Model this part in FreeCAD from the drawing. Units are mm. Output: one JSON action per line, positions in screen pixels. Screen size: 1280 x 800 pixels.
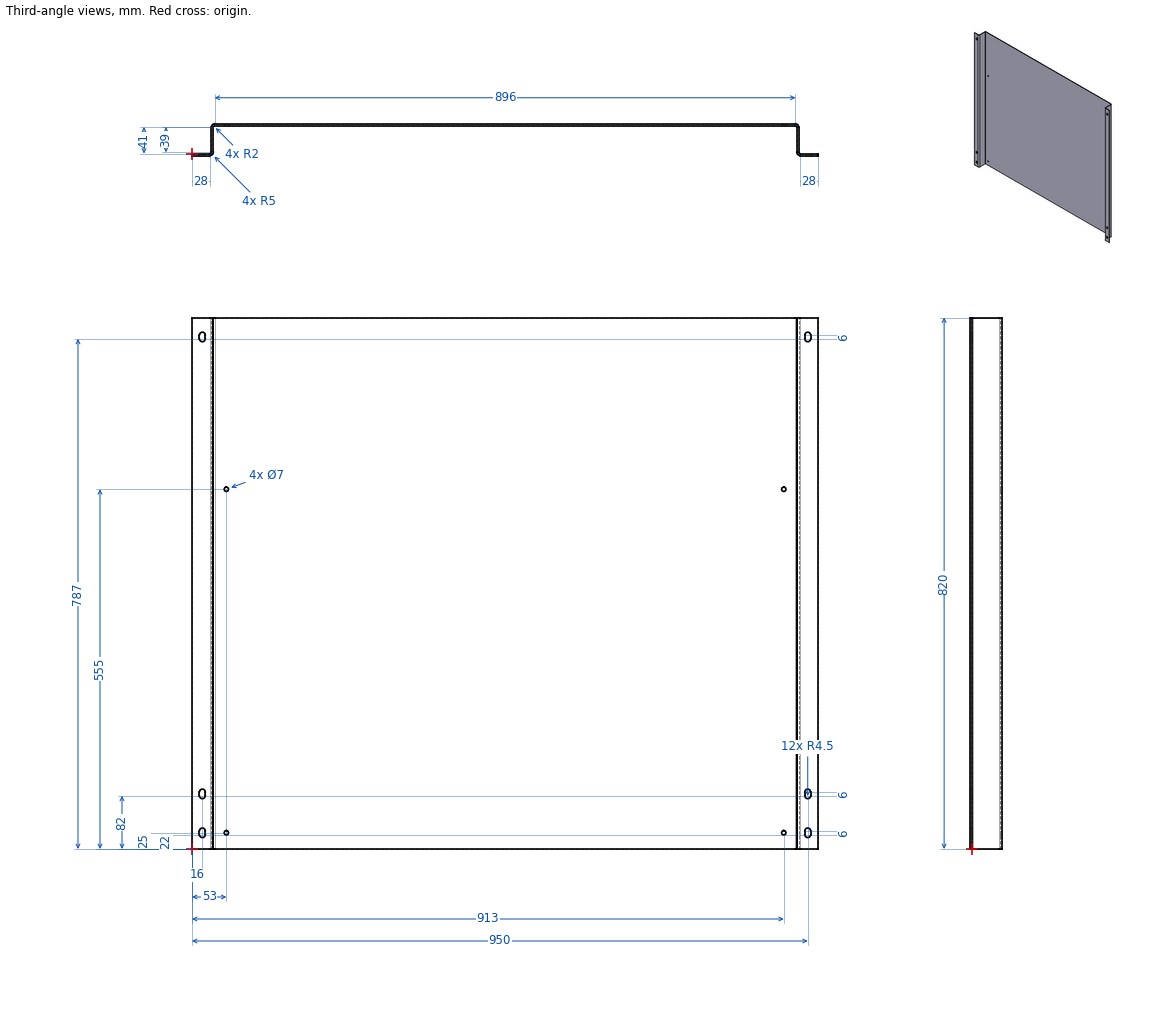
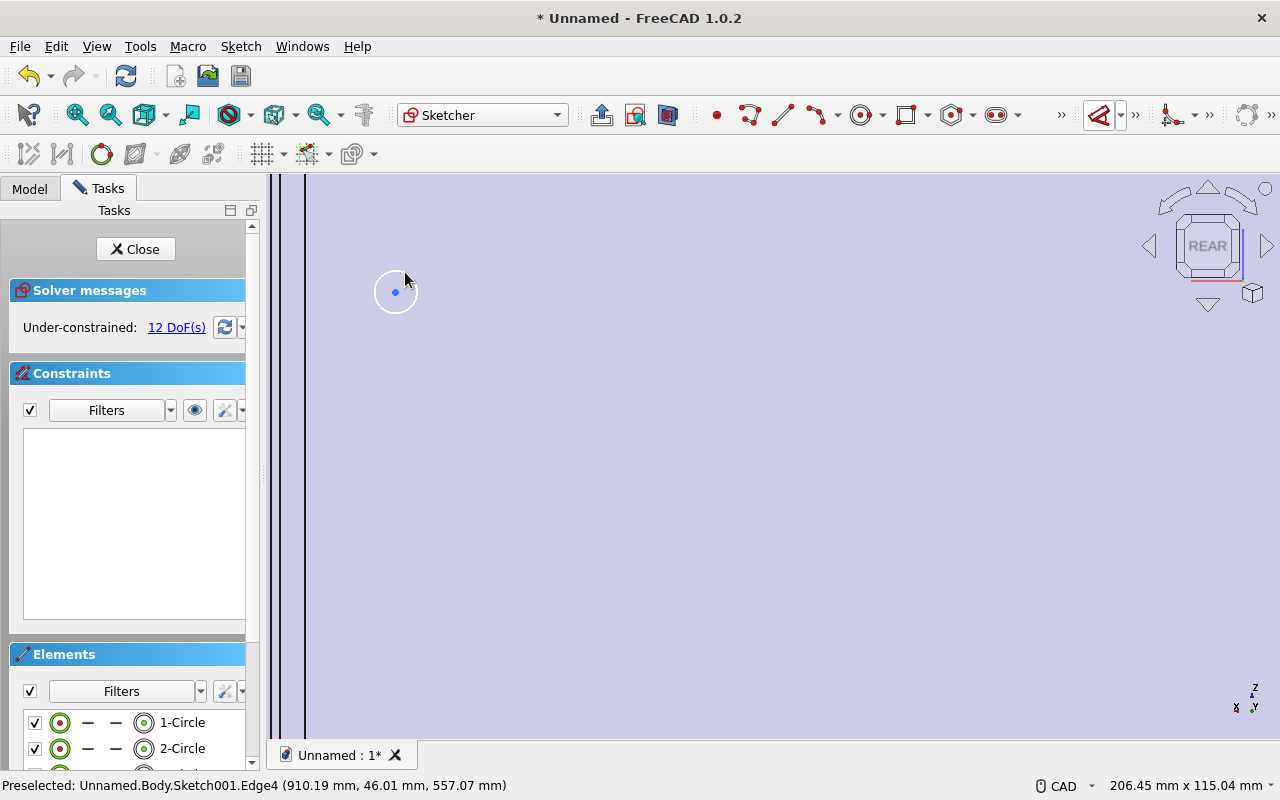
{"action": "scroll", "coordinate": [404, 271], "scroll_direction": "down", "scroll_amount": 10}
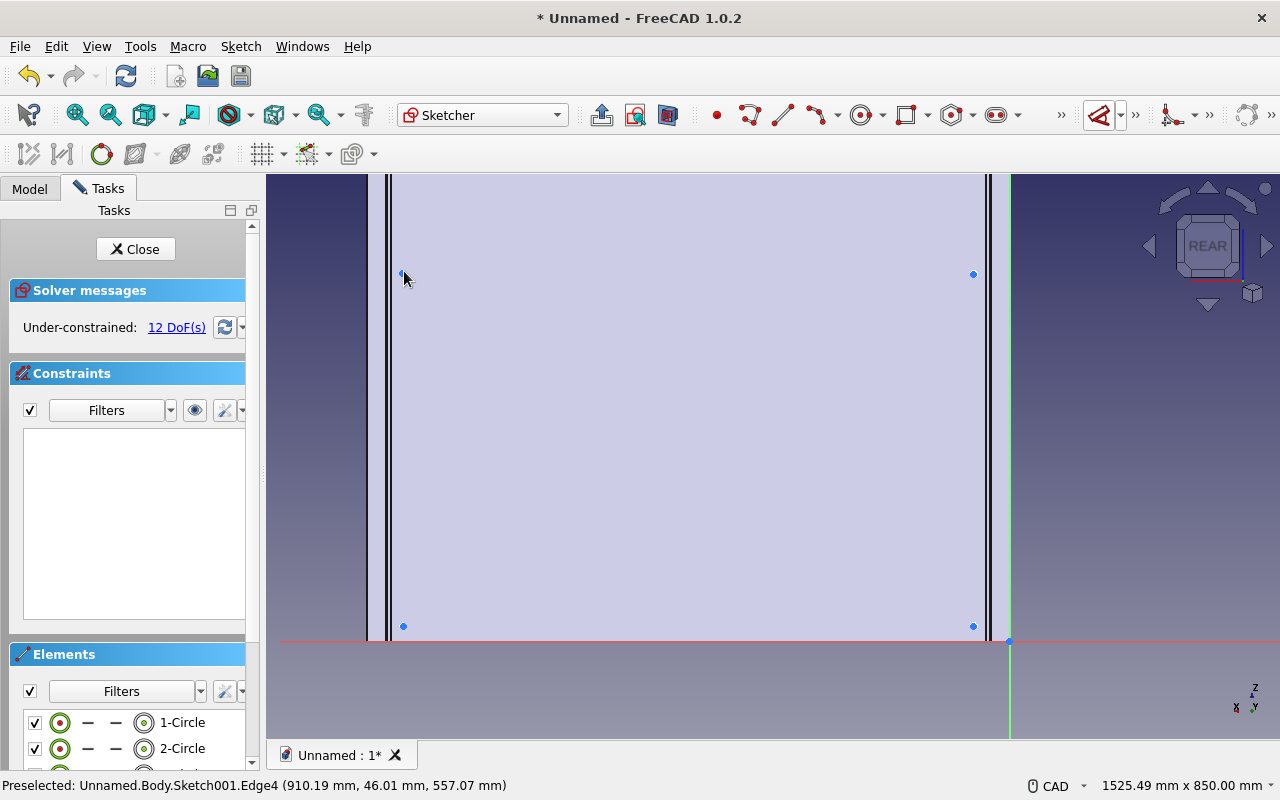
{"action": "scroll", "coordinate": [976, 272], "scroll_direction": "up", "scroll_amount": 8}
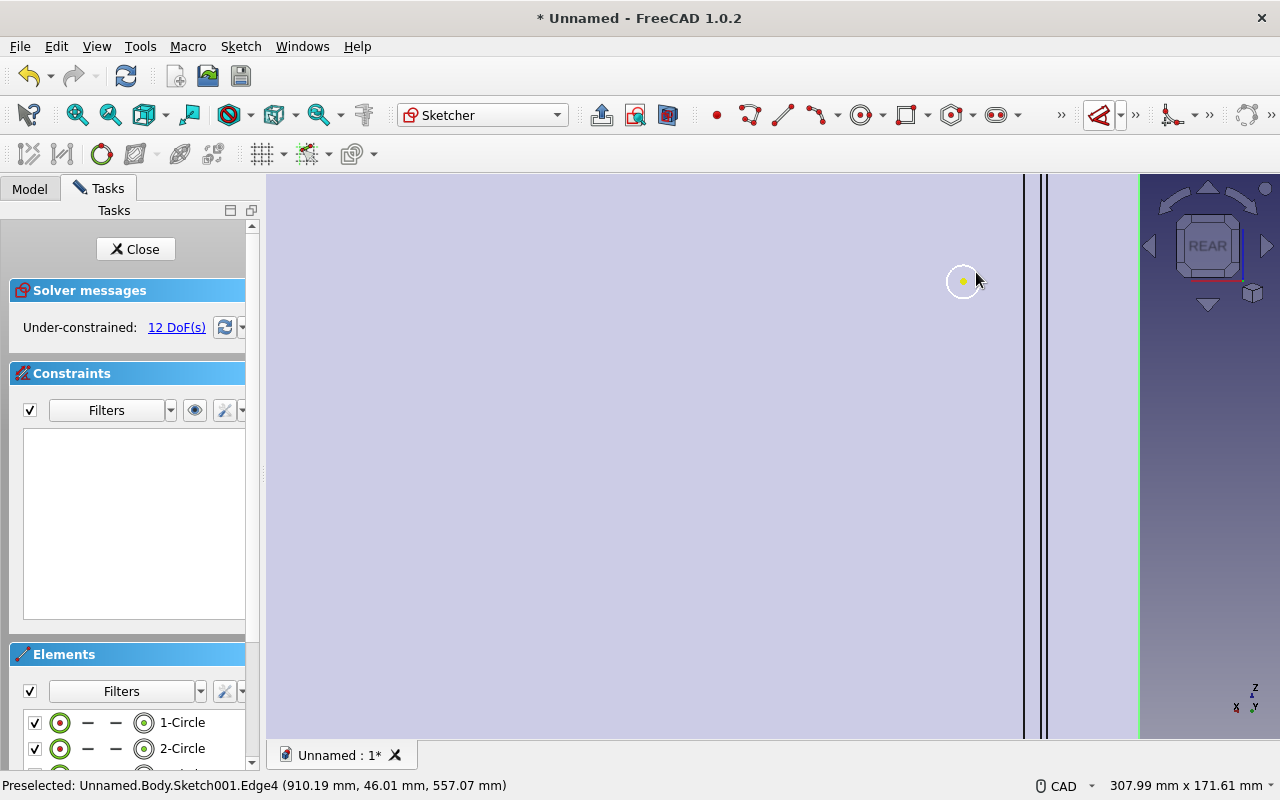
{"action": "left_click", "coordinate": [975, 270]}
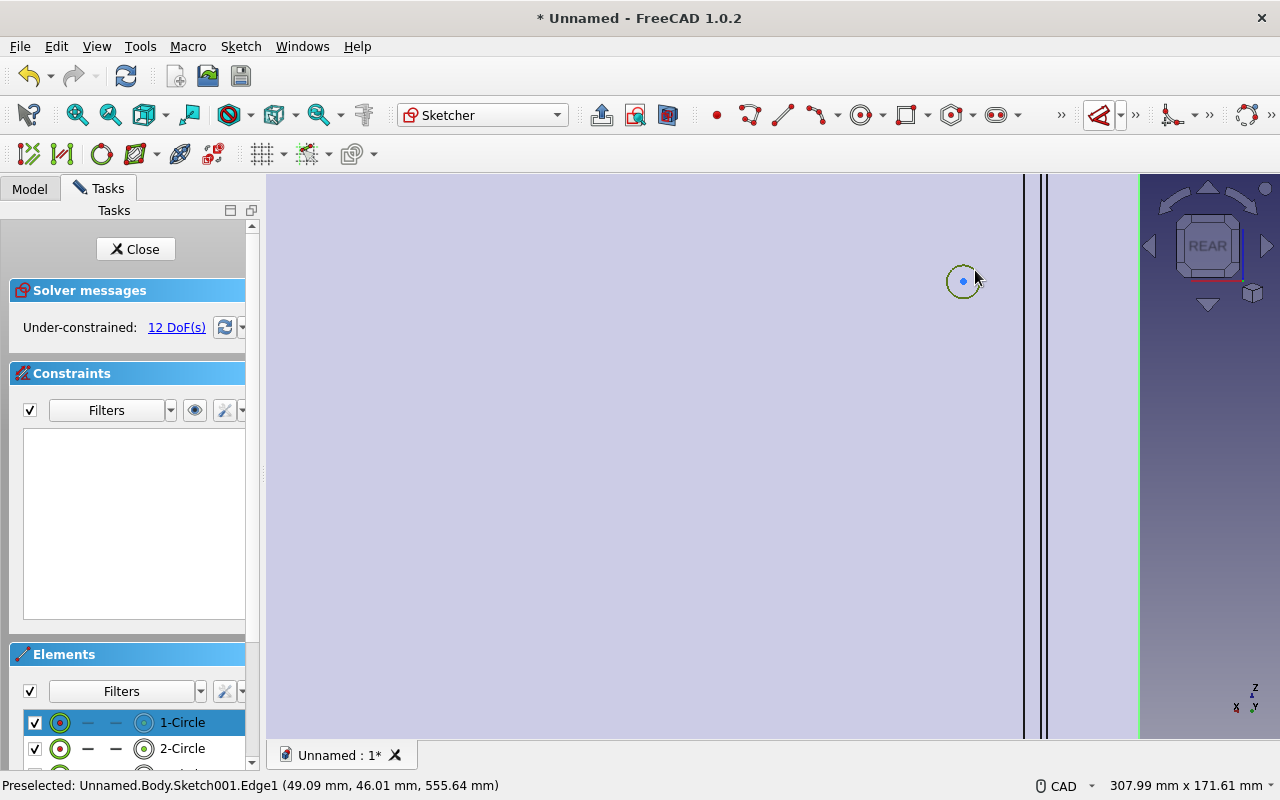
{"action": "scroll", "coordinate": [976, 272], "scroll_direction": "down", "scroll_amount": 8}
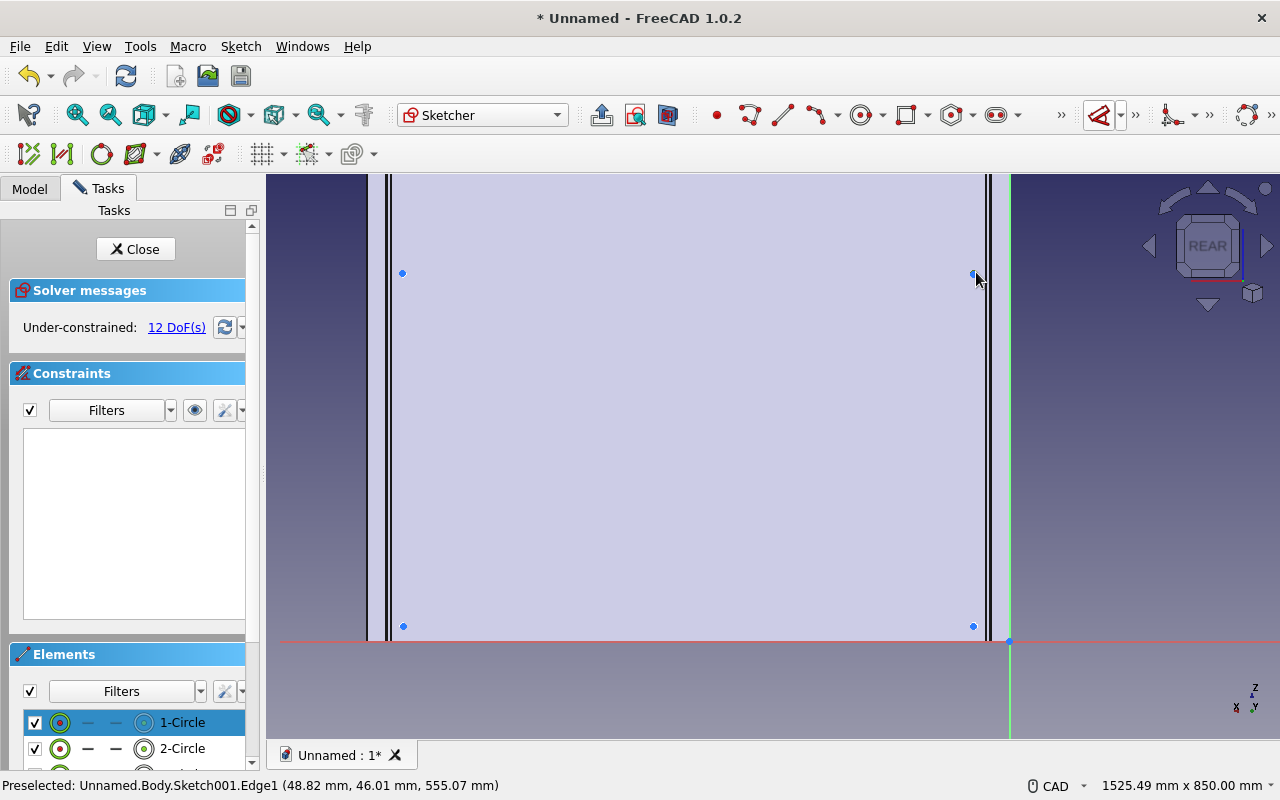
{"action": "scroll", "coordinate": [976, 624], "scroll_direction": "up", "scroll_amount": 8}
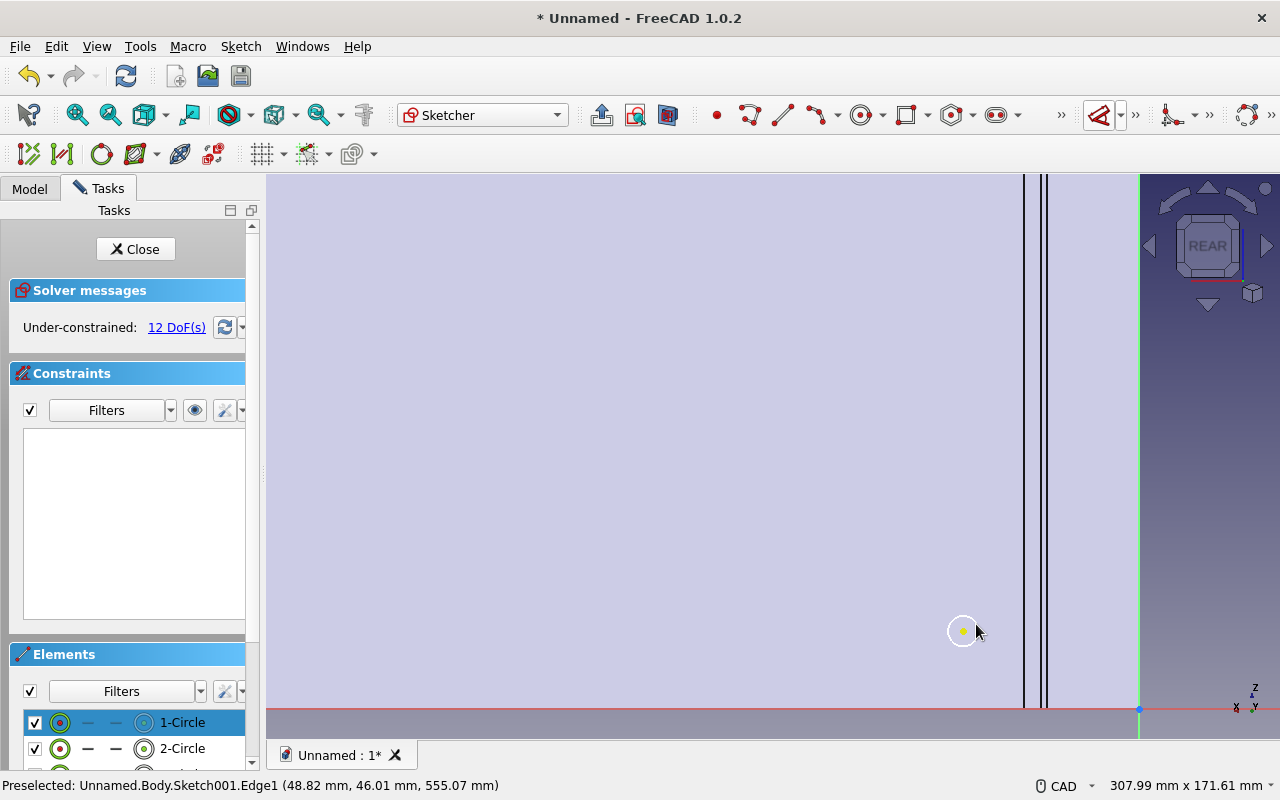
{"action": "left_click", "coordinate": [974, 620]}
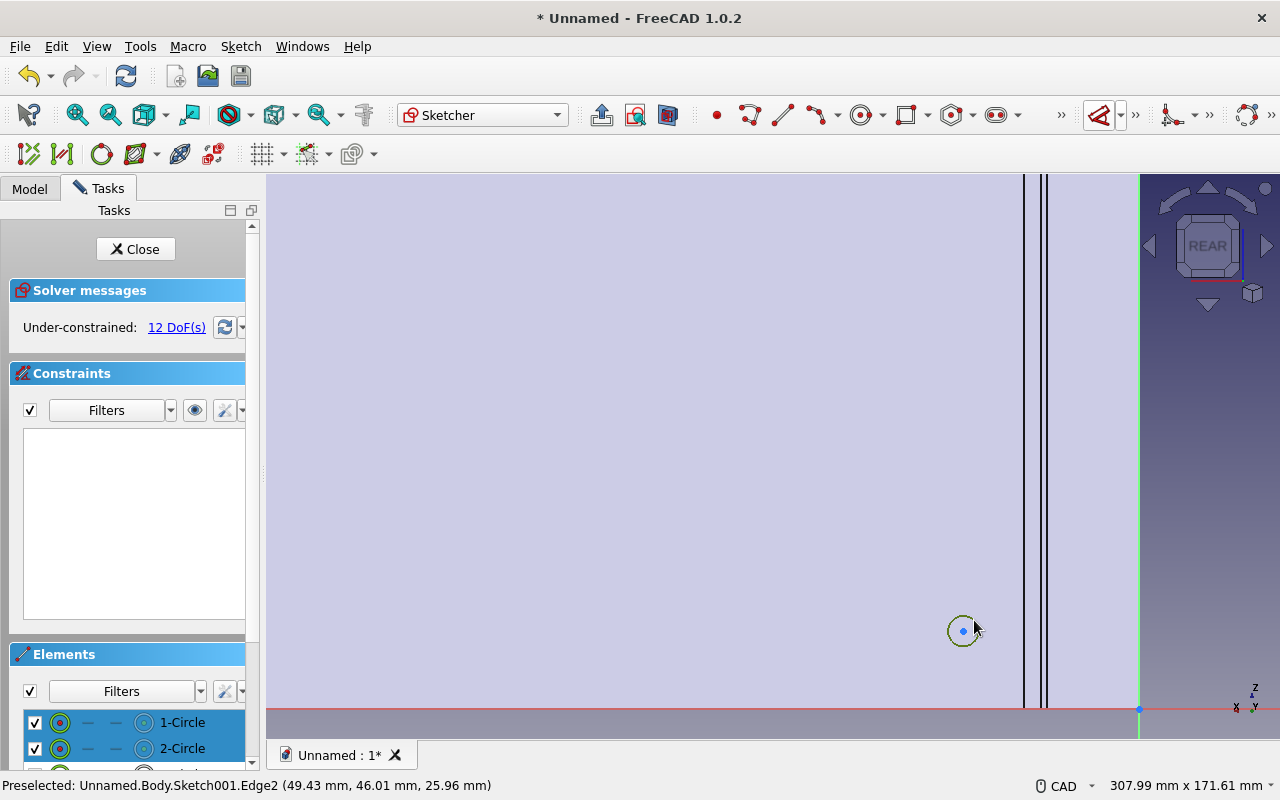
{"action": "scroll", "coordinate": [976, 625], "scroll_direction": "down", "scroll_amount": 8}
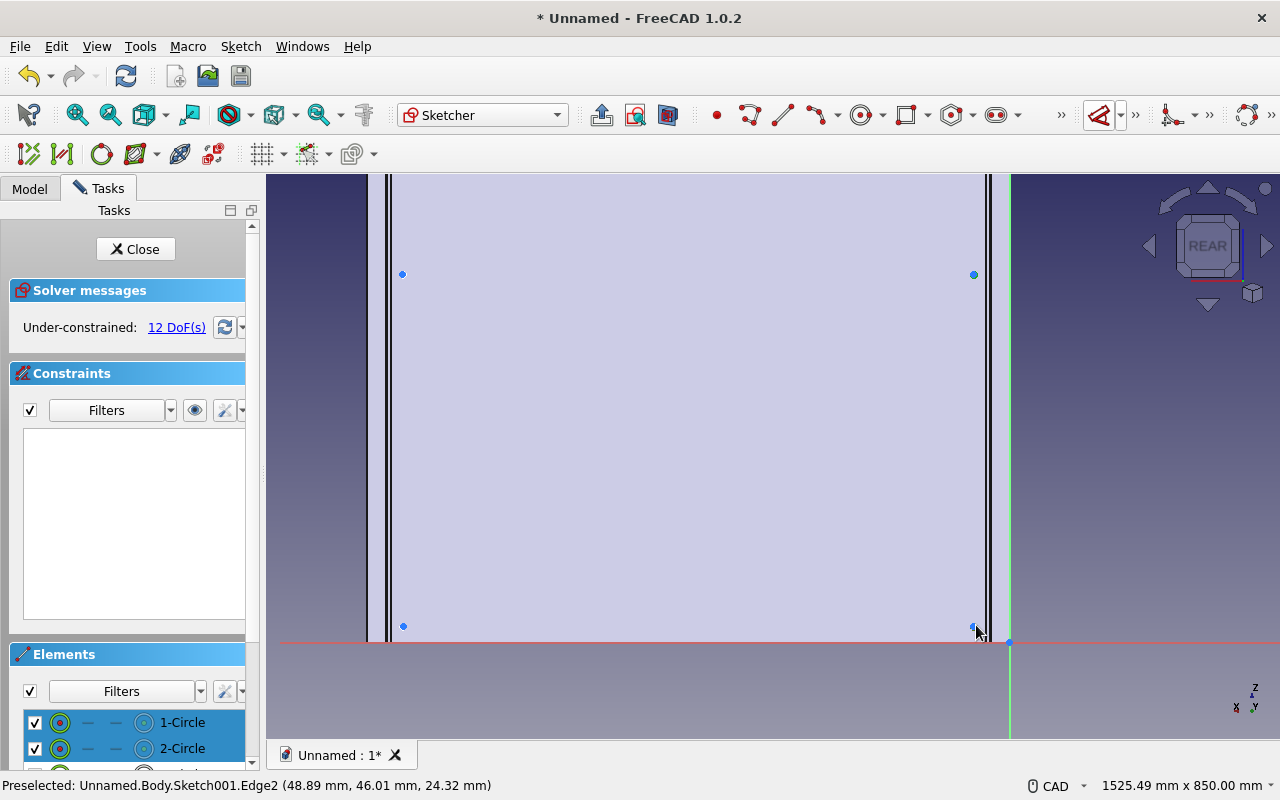
{"action": "scroll", "coordinate": [405, 625], "scroll_direction": "up", "scroll_amount": 9}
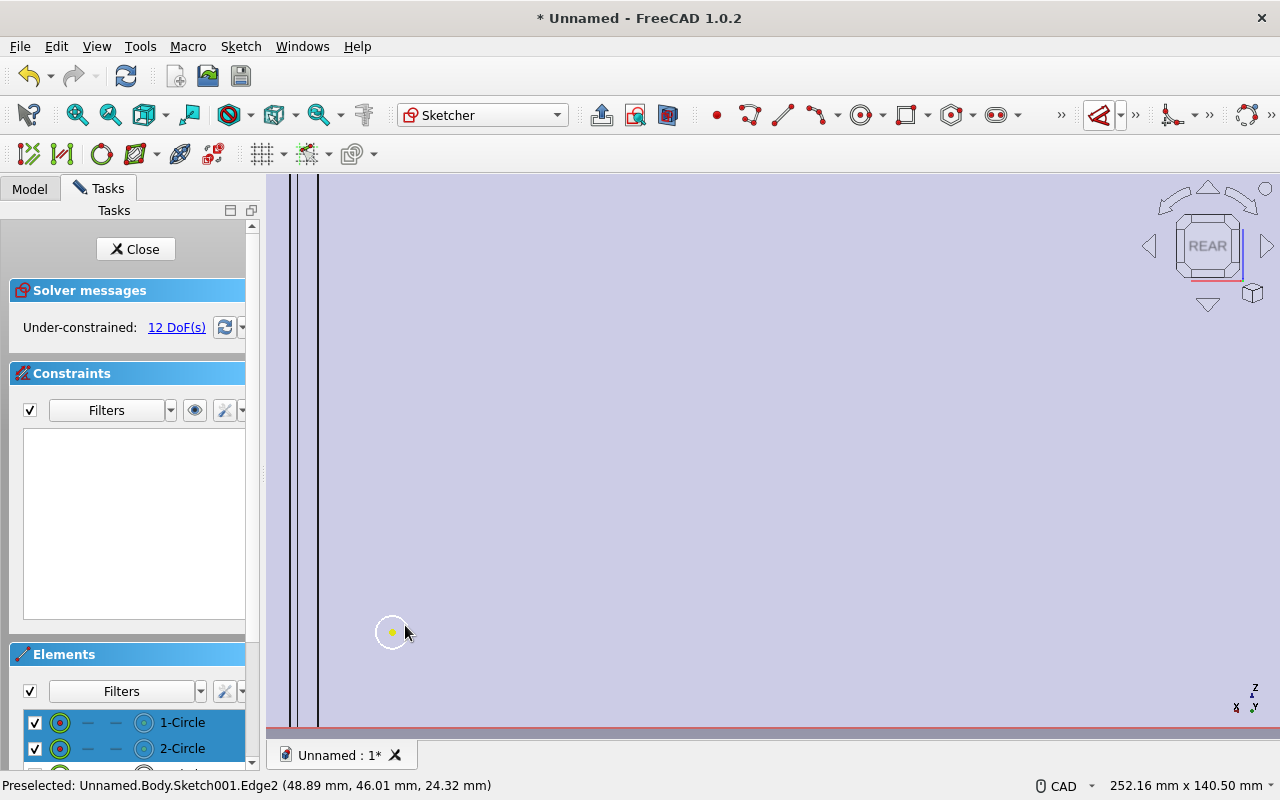
{"action": "left_click", "coordinate": [404, 621]}